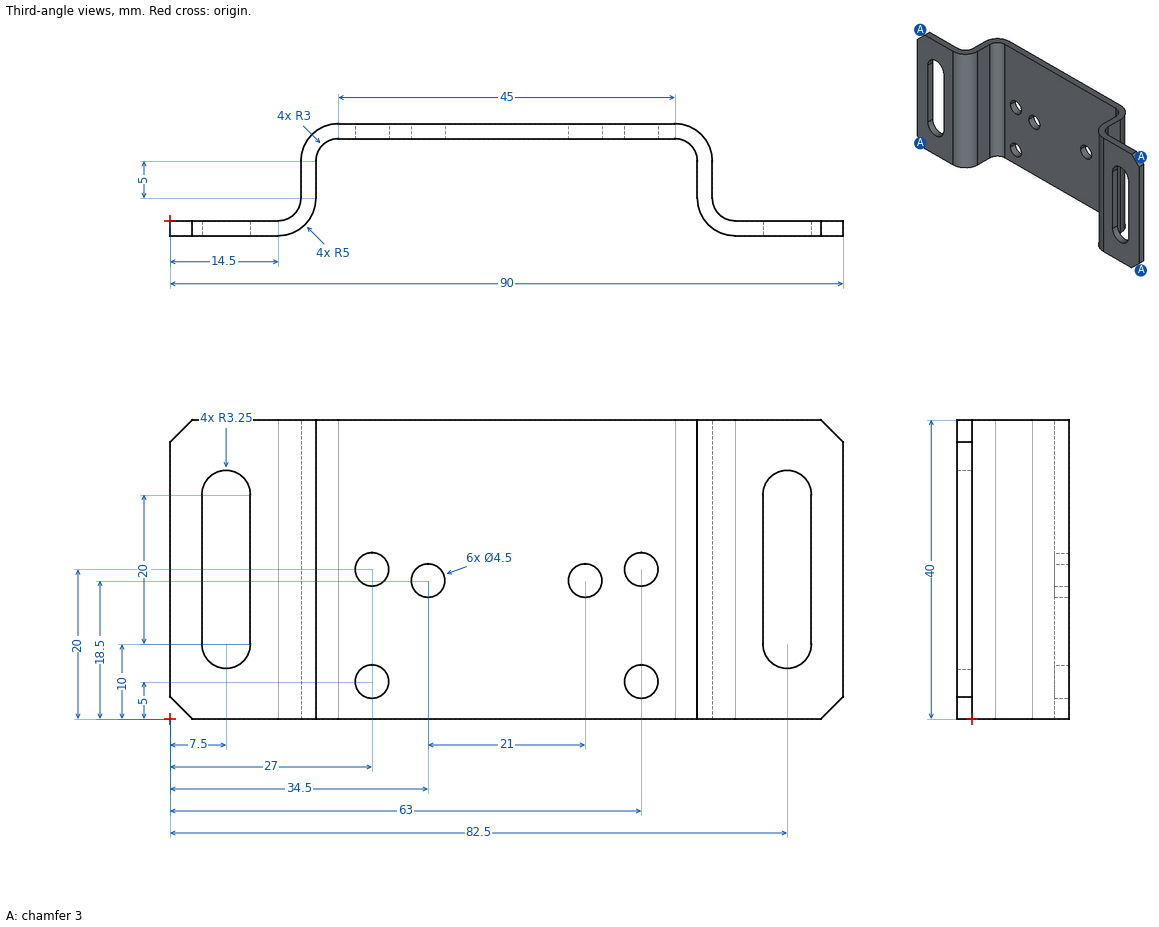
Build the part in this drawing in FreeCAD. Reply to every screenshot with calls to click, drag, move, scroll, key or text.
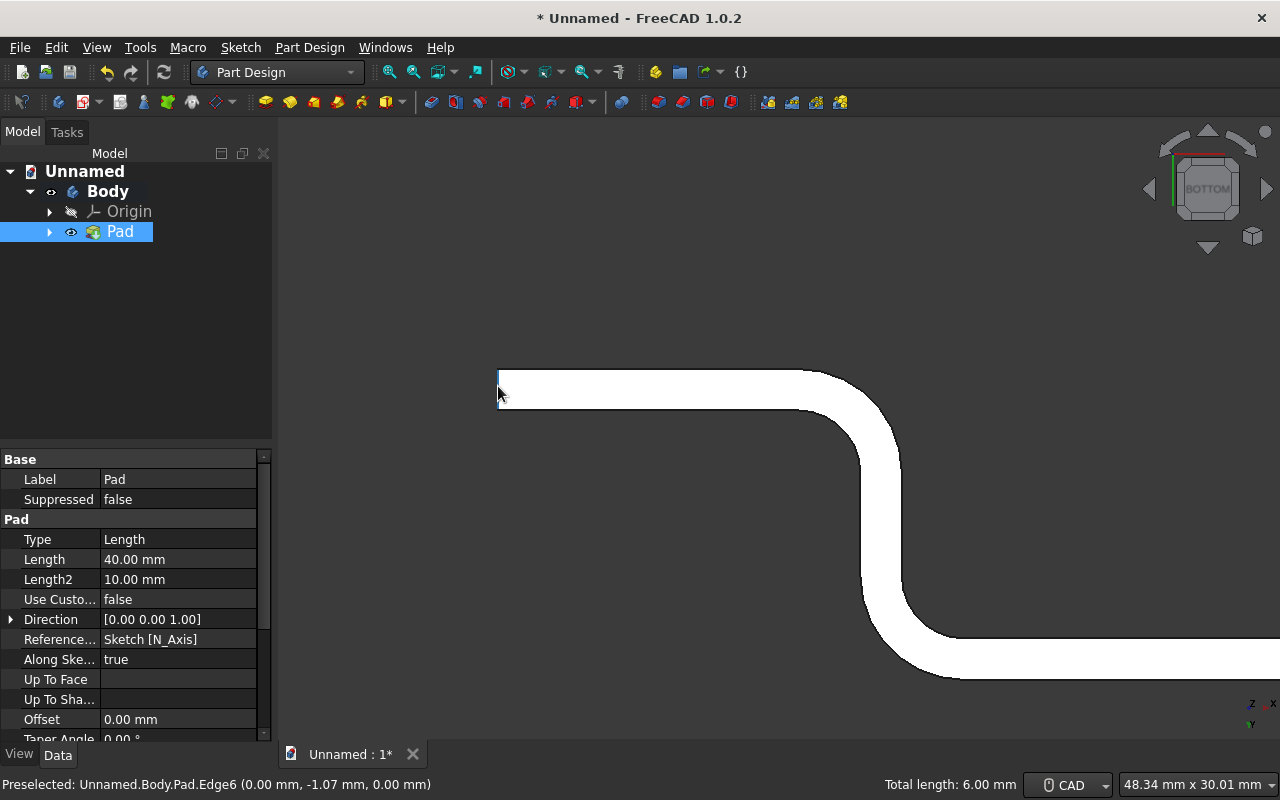
click(498, 389, ctrl)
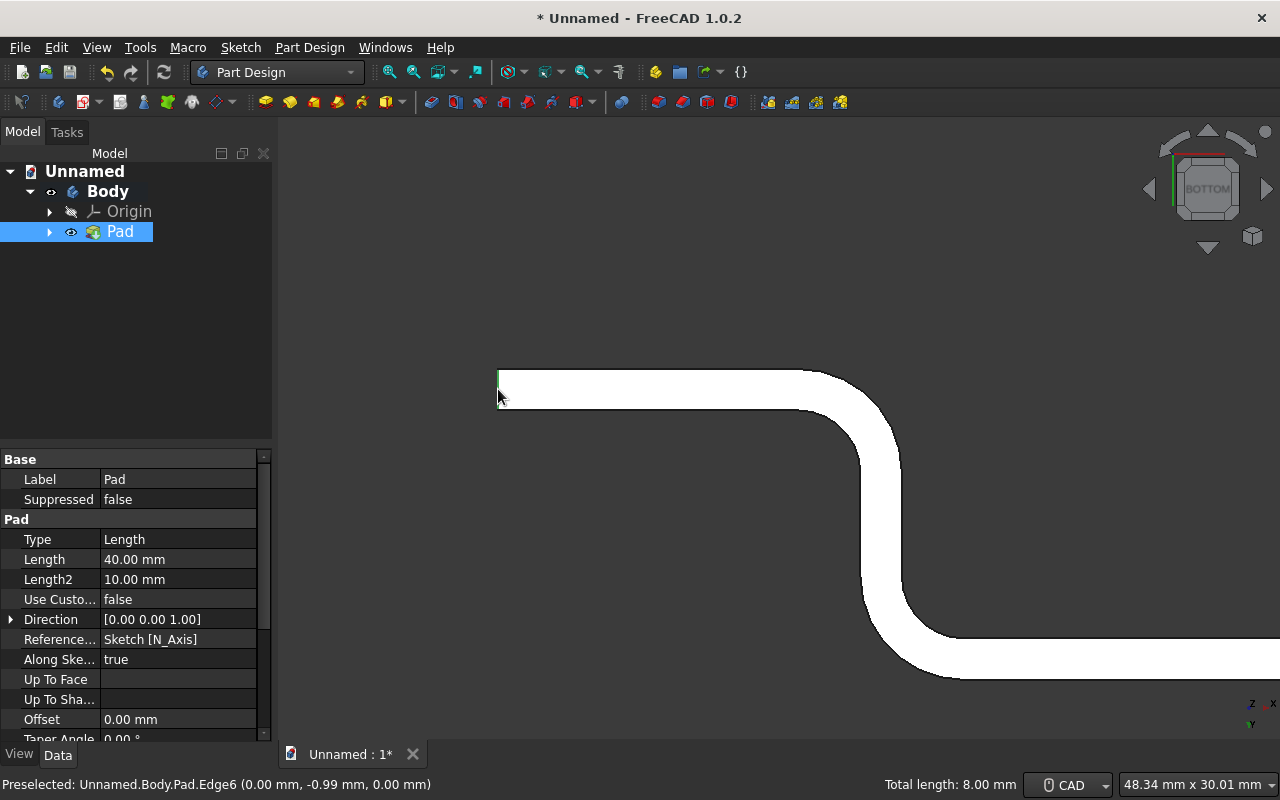
click(684, 102)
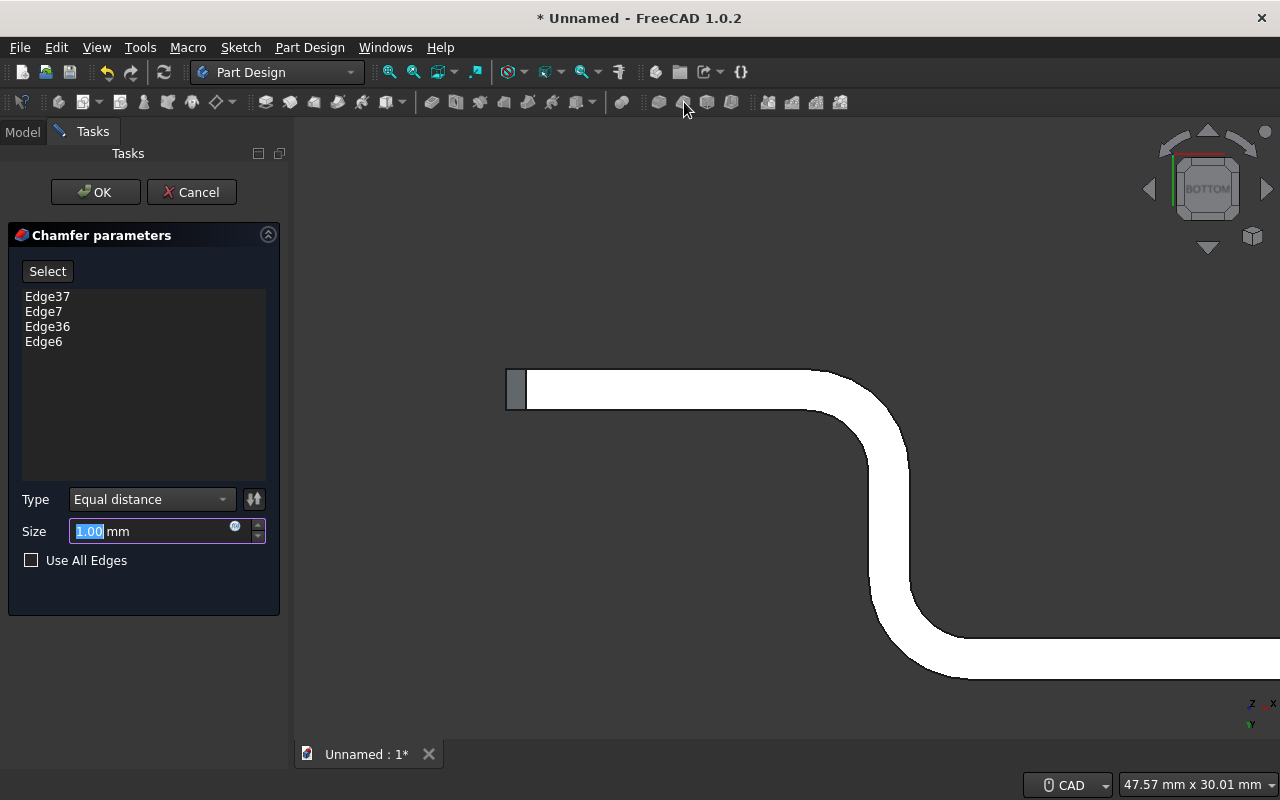
text(3)
key(Tab)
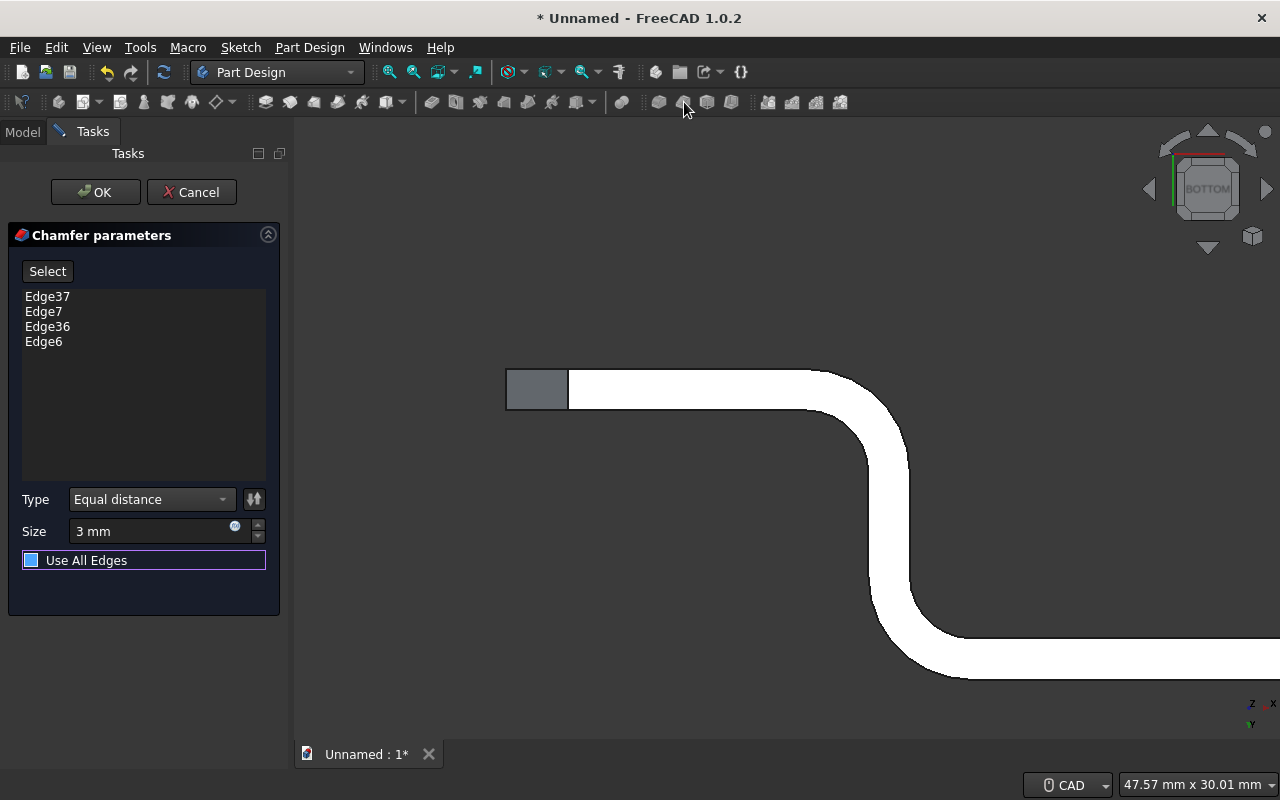
click(96, 192)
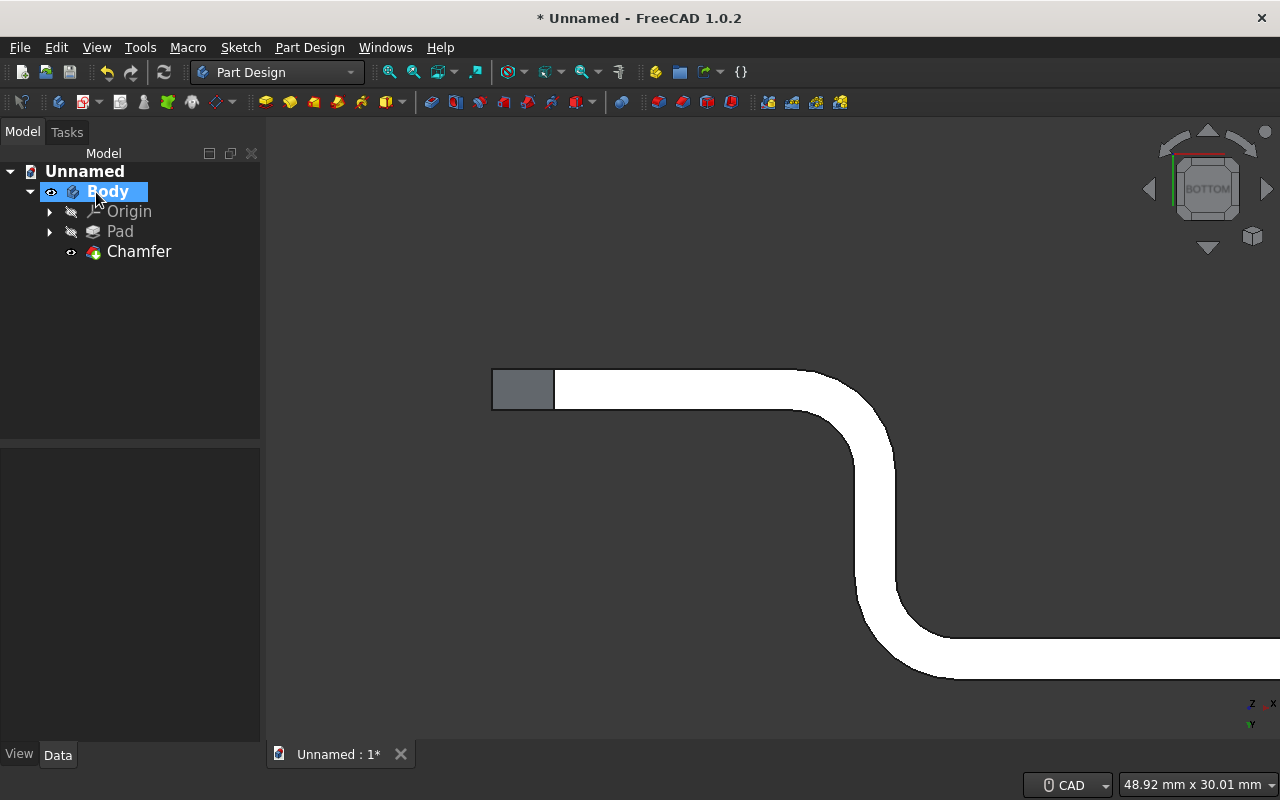
key(v)
key(f)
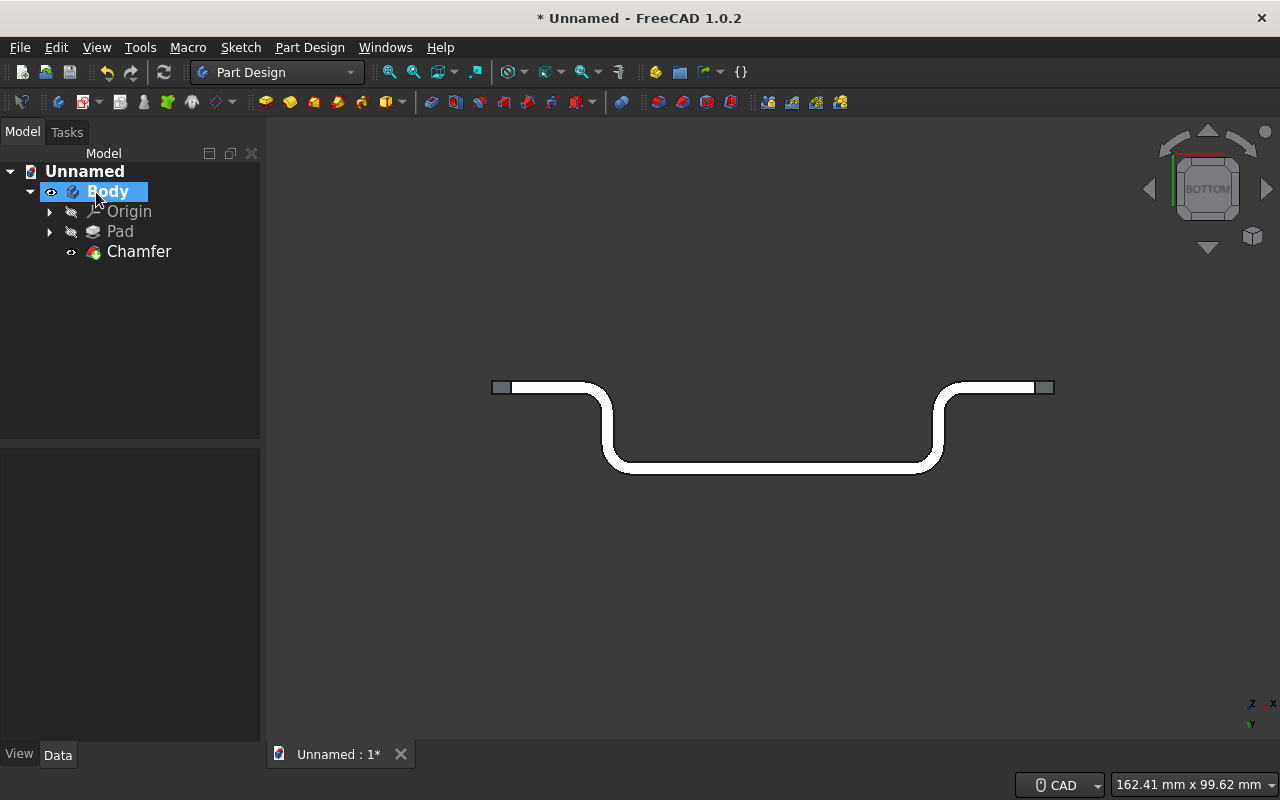
key(4)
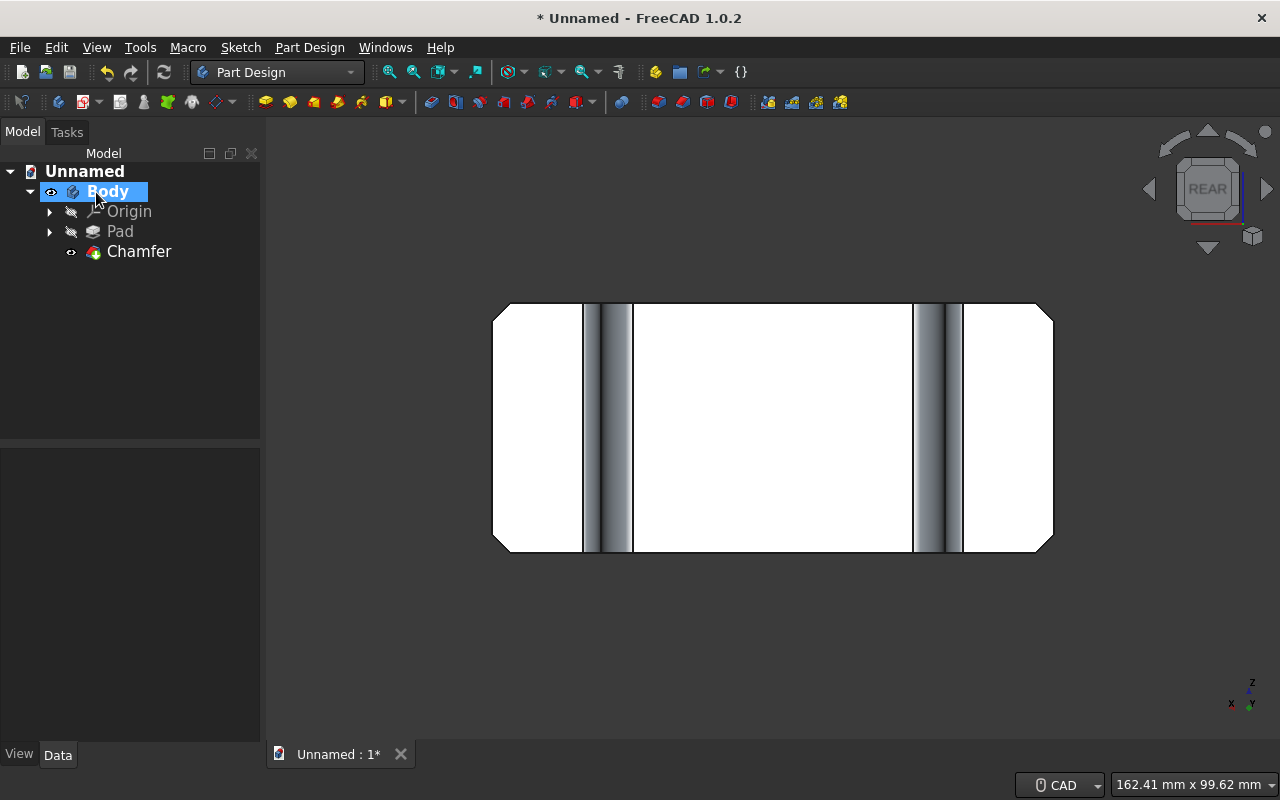
click(537, 356)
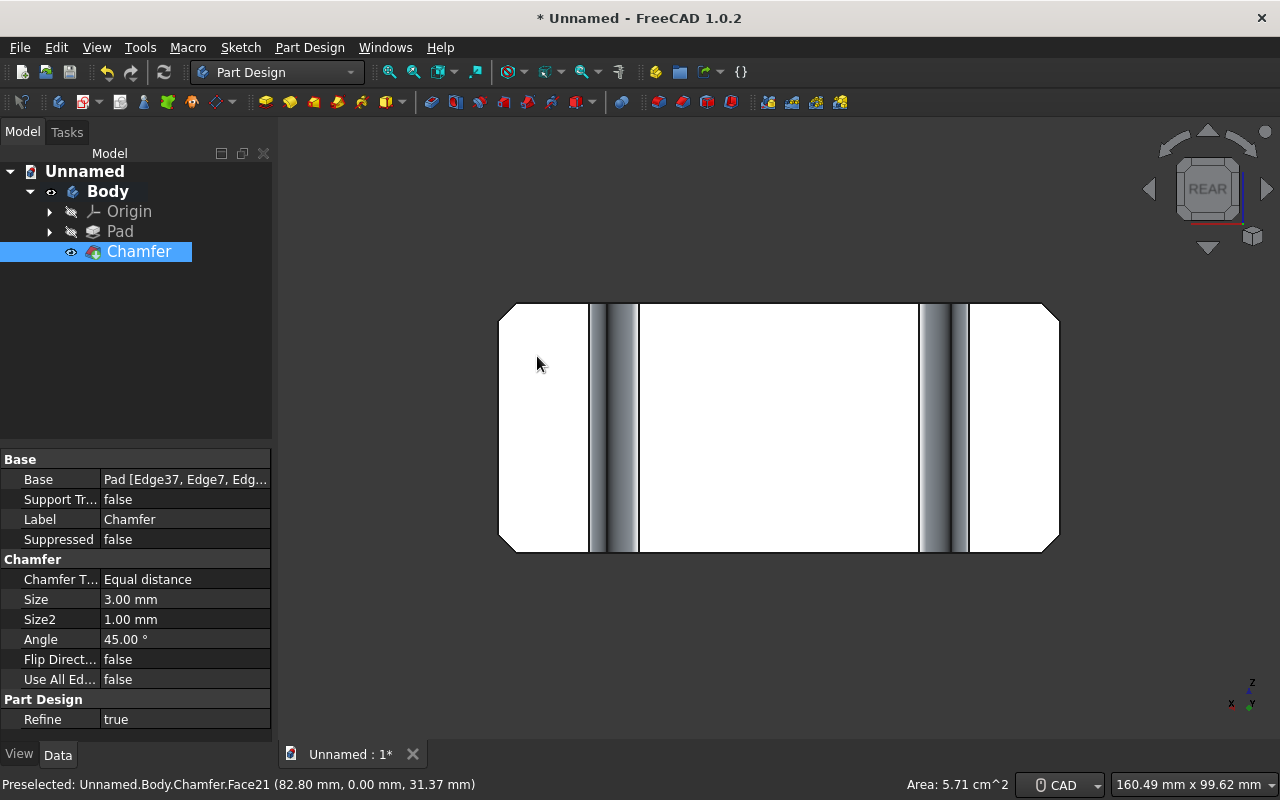
click(84, 102)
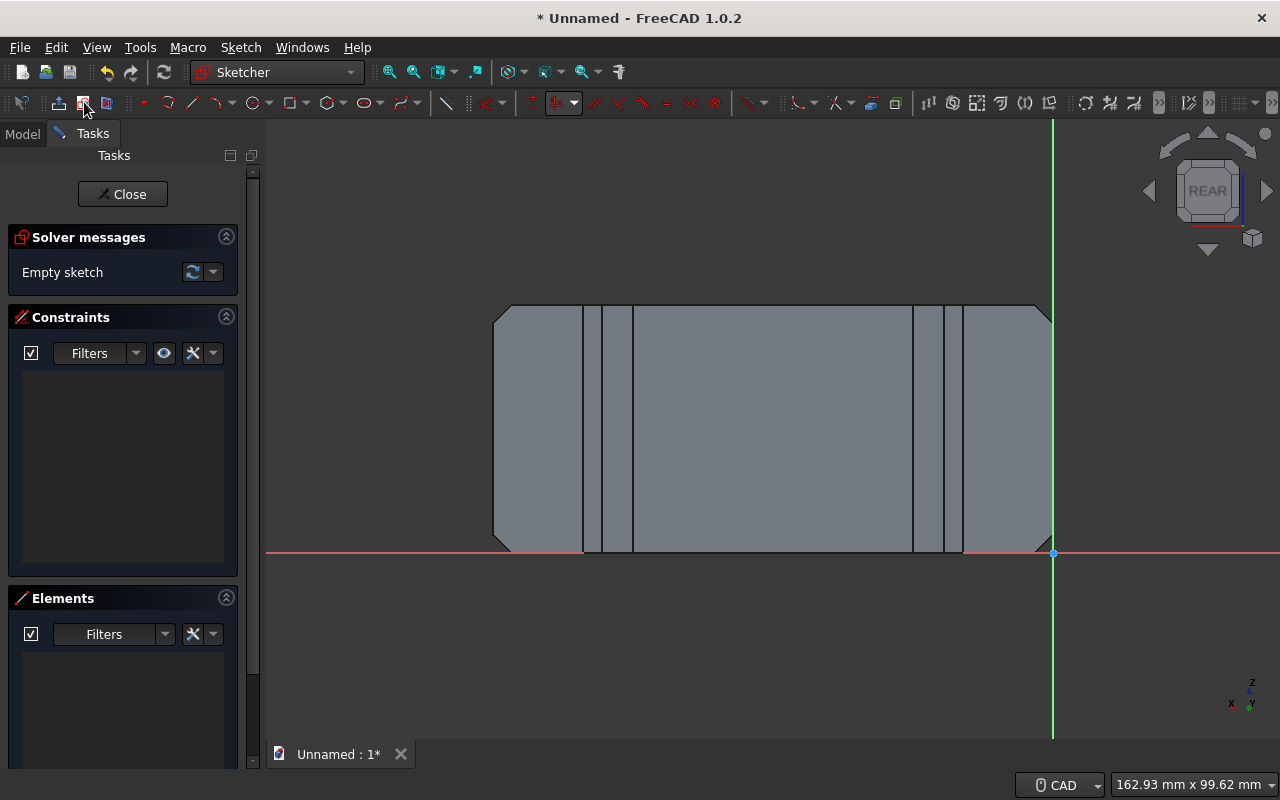
key(g)
key(s)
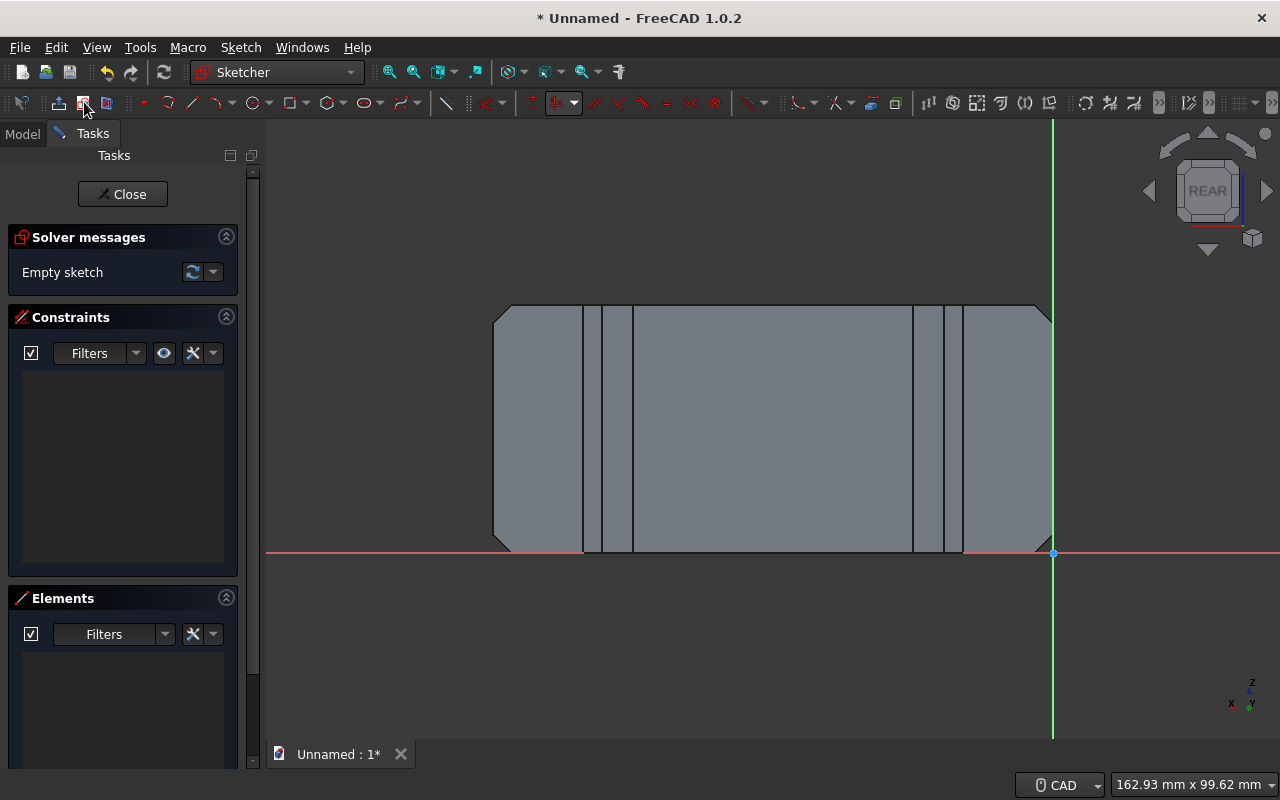
click(1006, 491)